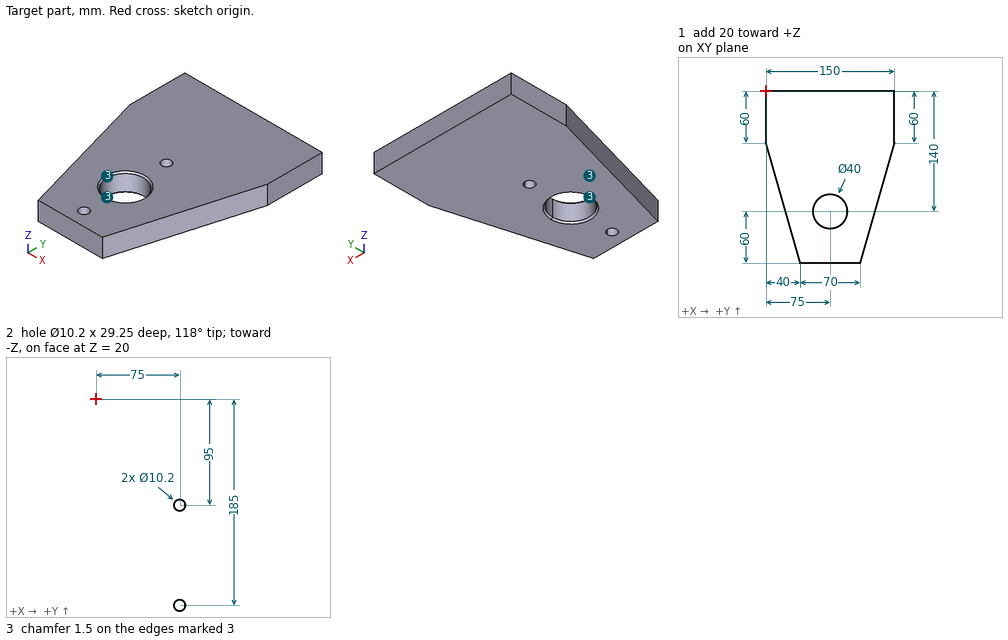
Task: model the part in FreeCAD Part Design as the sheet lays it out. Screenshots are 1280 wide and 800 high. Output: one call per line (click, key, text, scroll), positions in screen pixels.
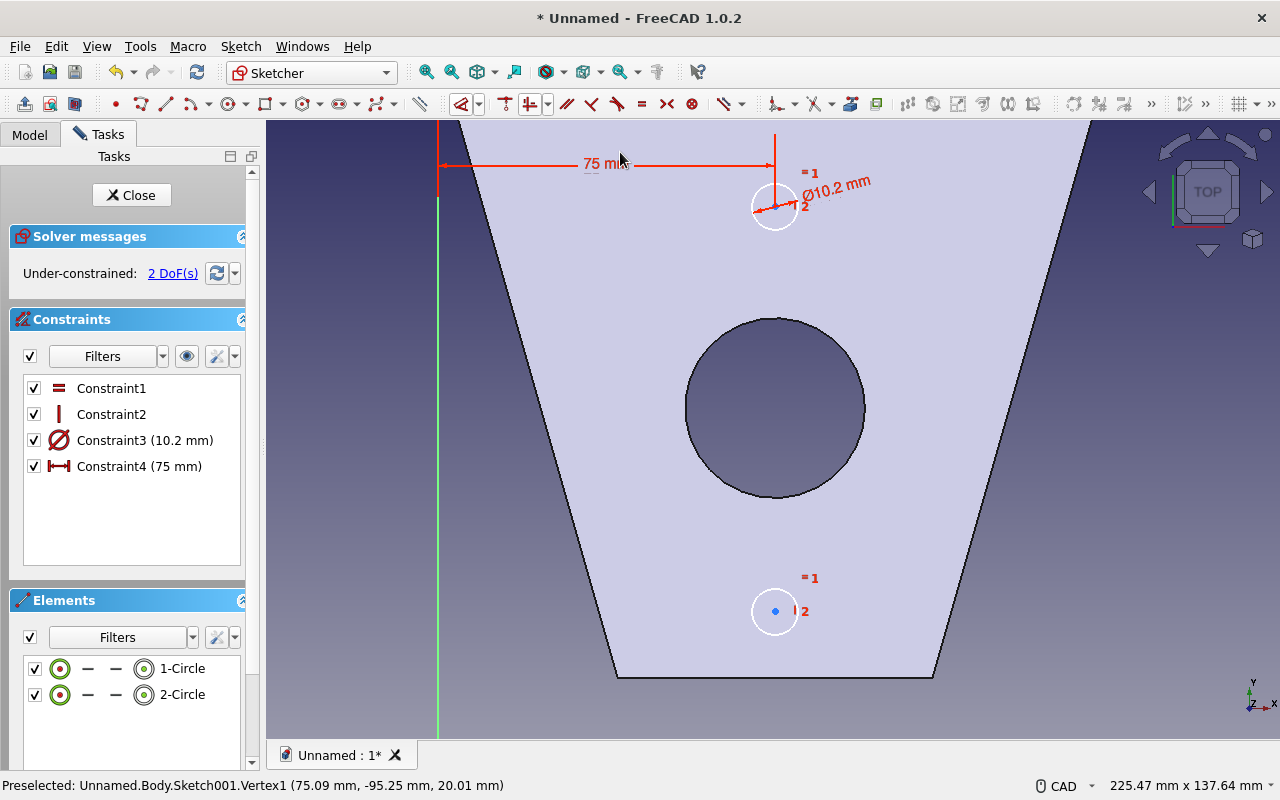
click(775, 207)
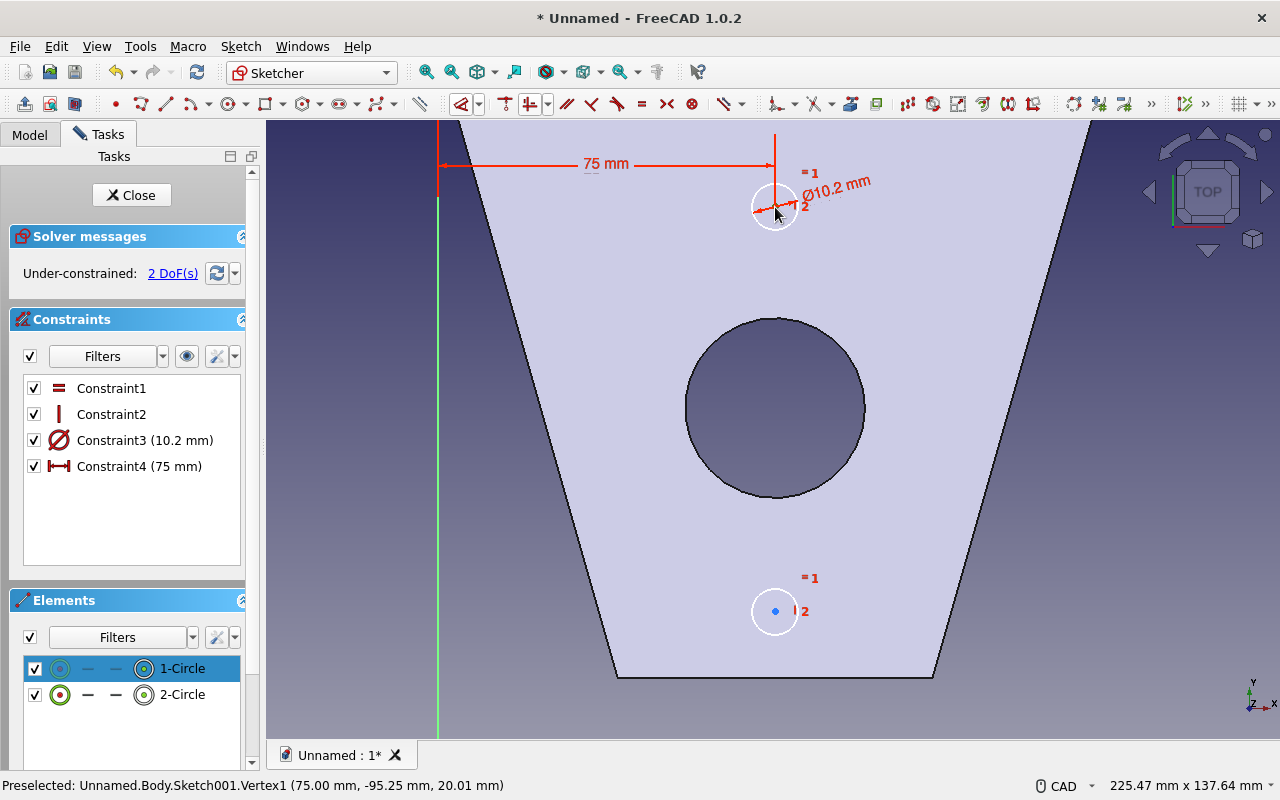
click(478, 104)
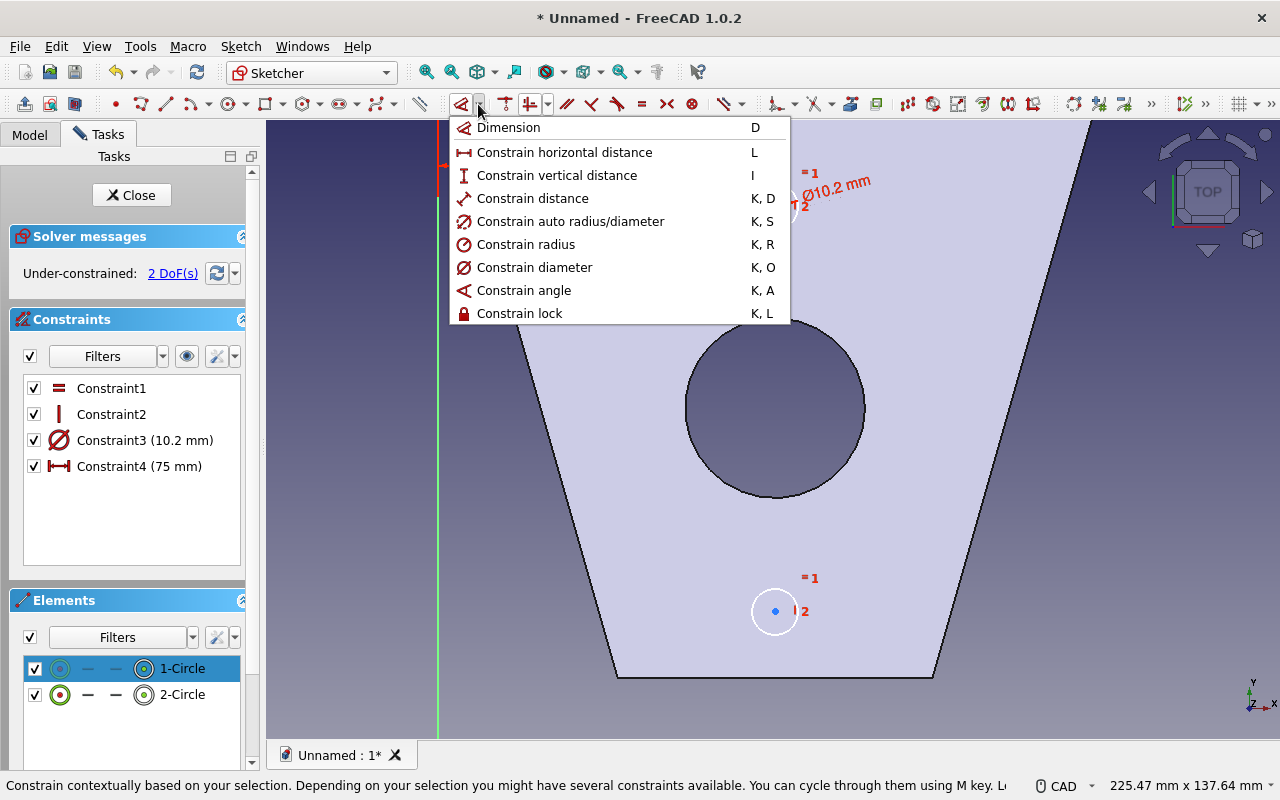
click(620, 176)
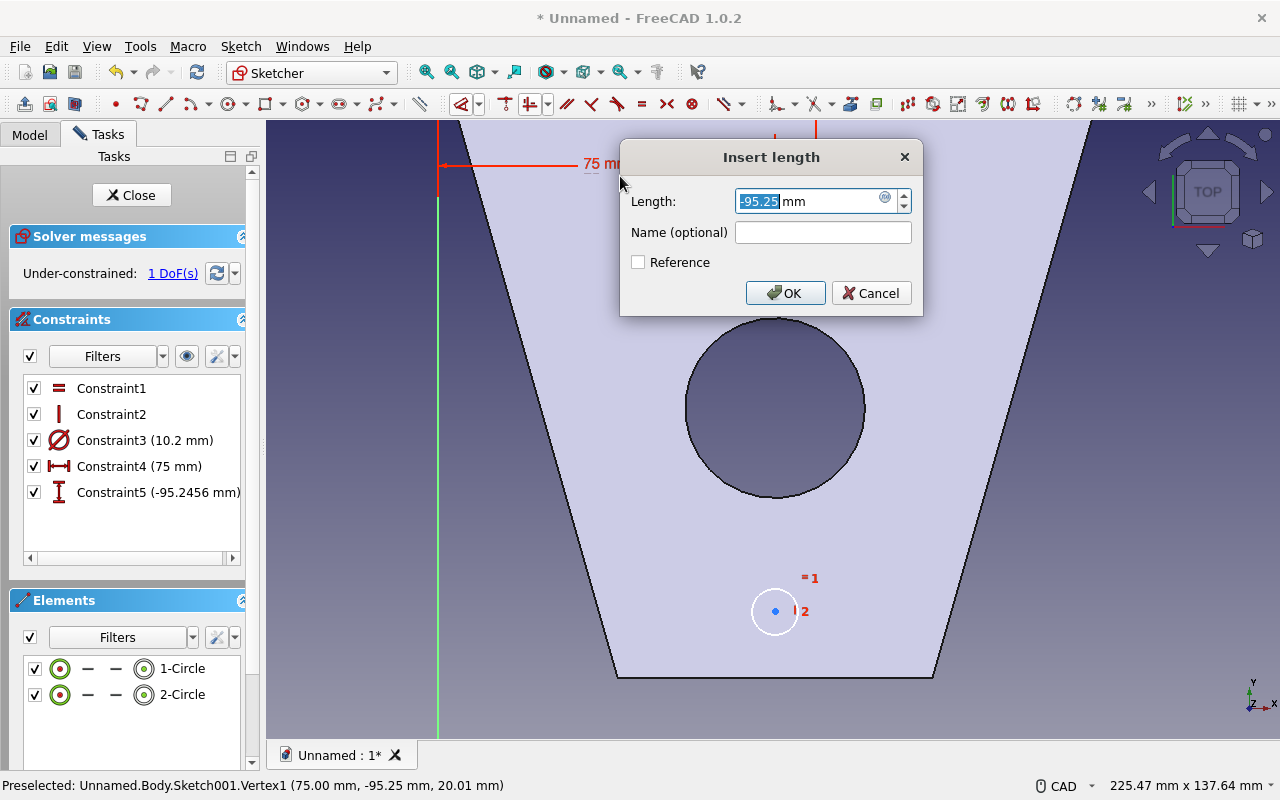
text(-95)
key(Return)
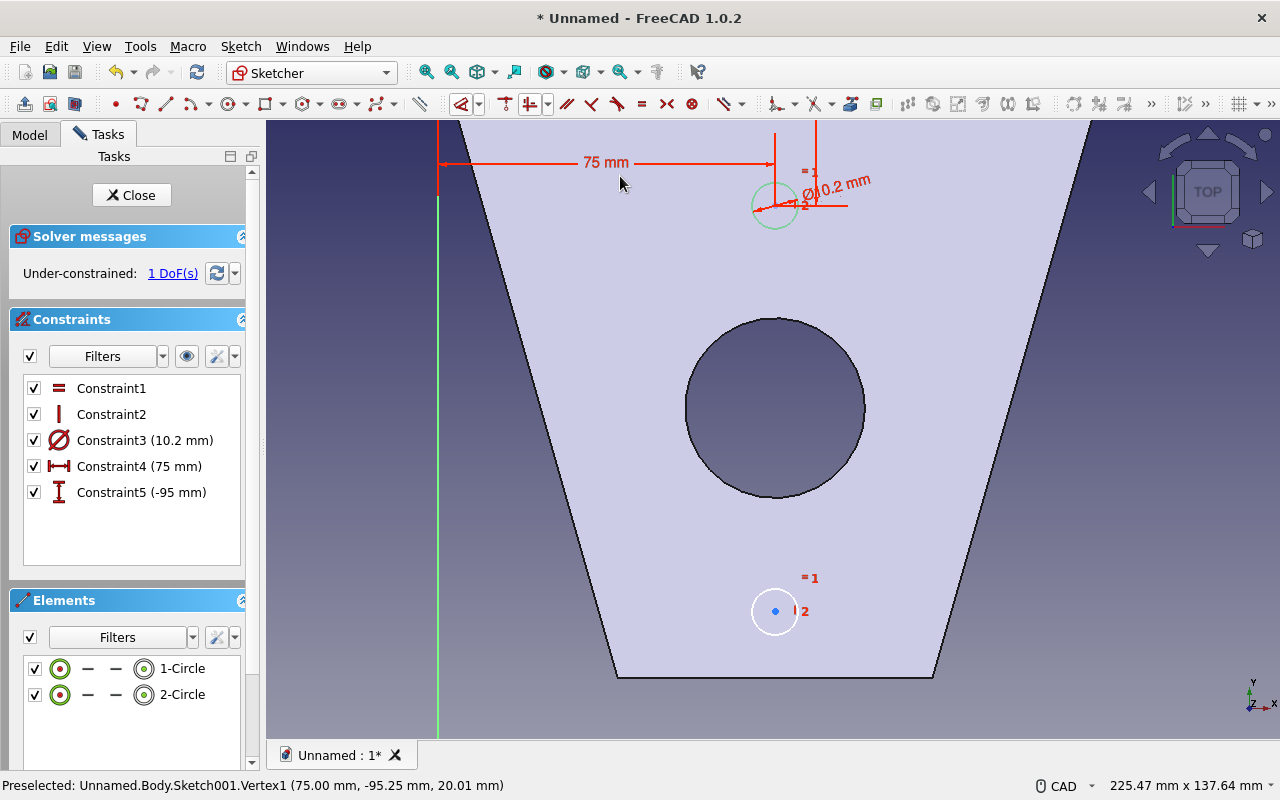
click(775, 612)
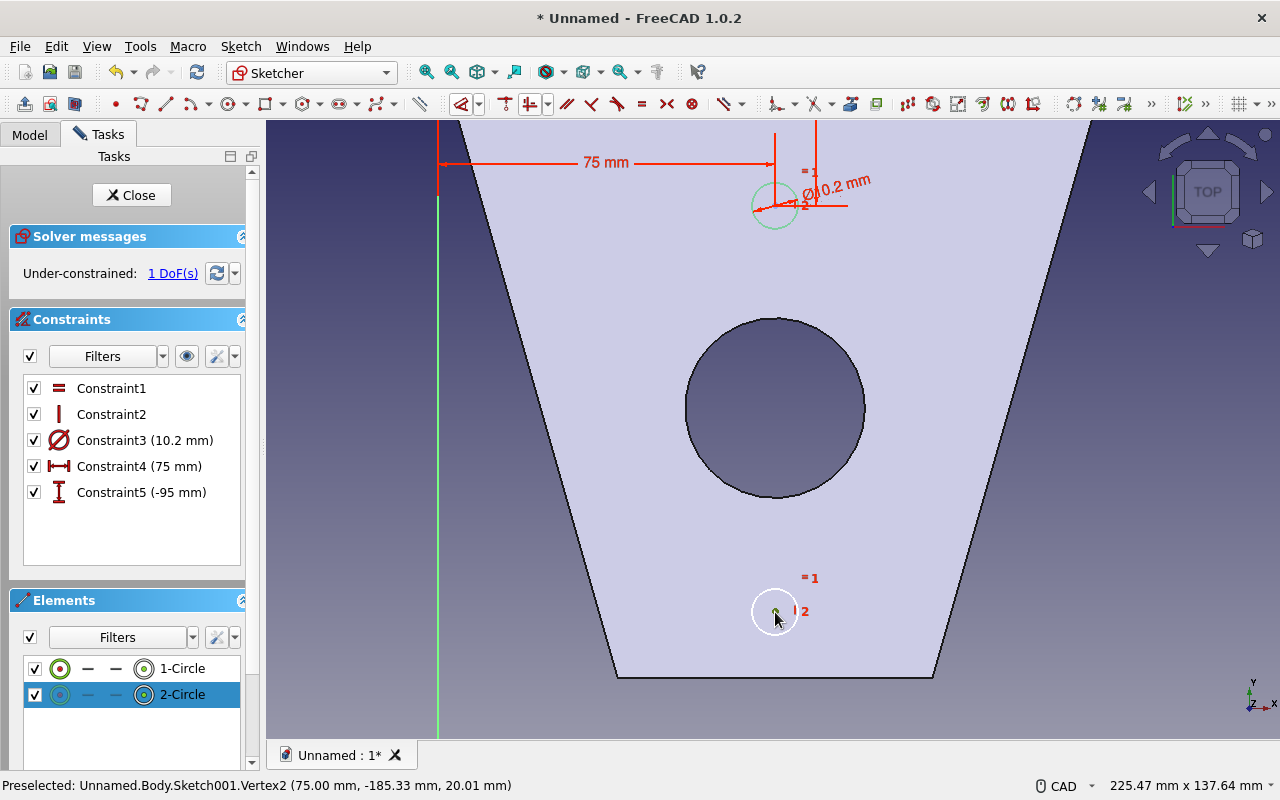
key(i)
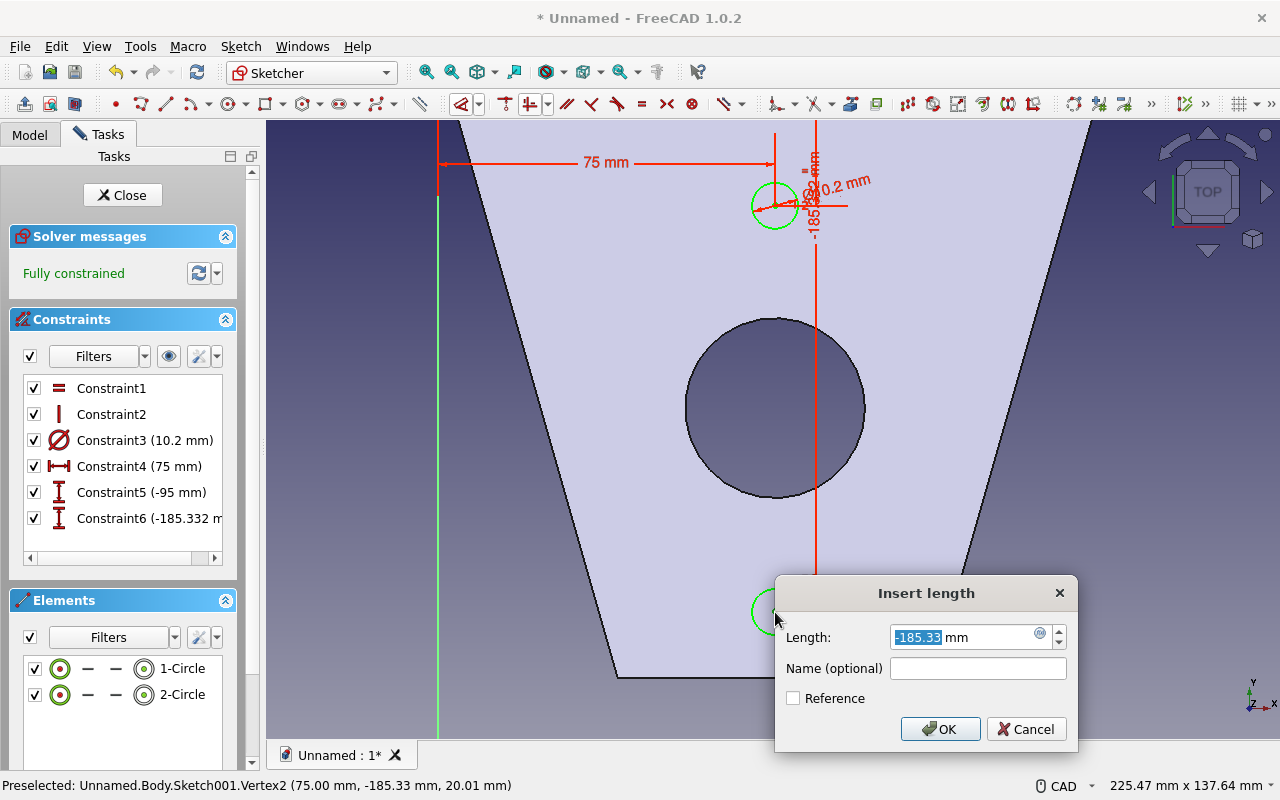
text(-185)
key(Return)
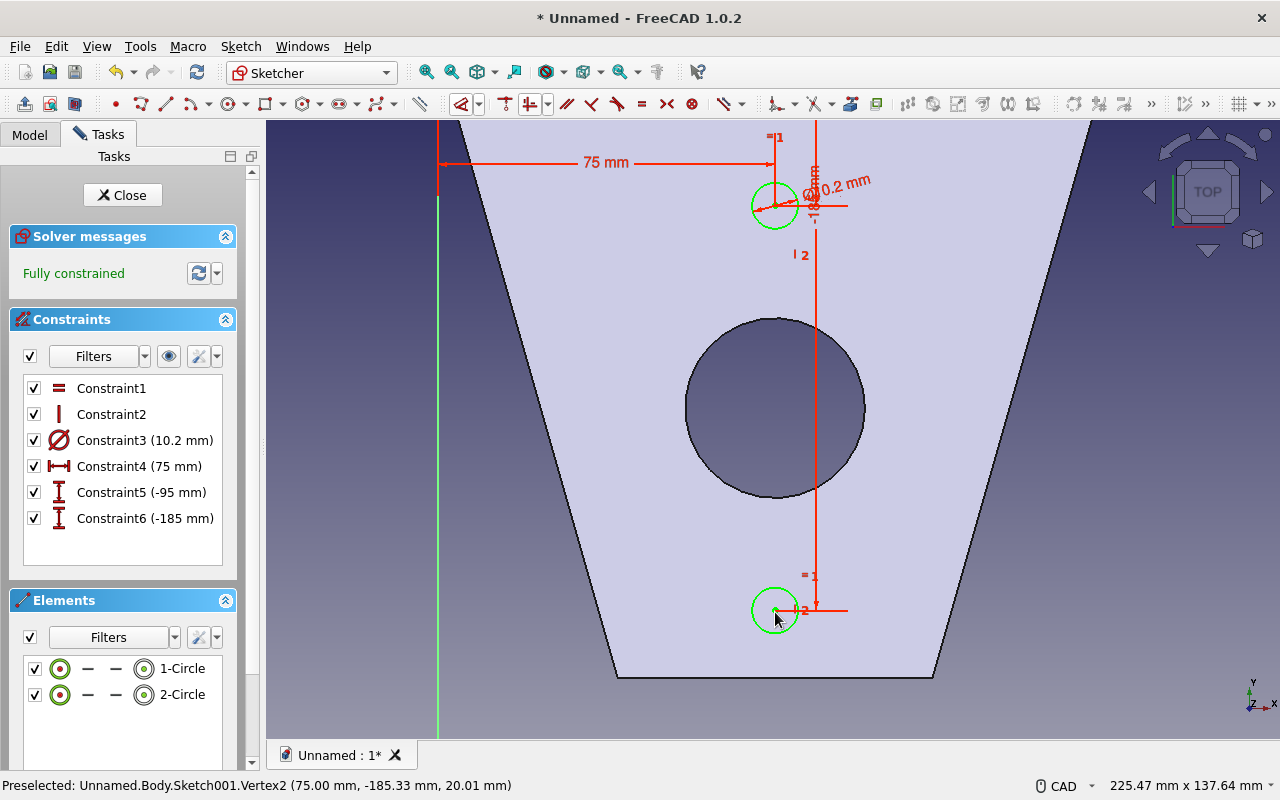
click(123, 195)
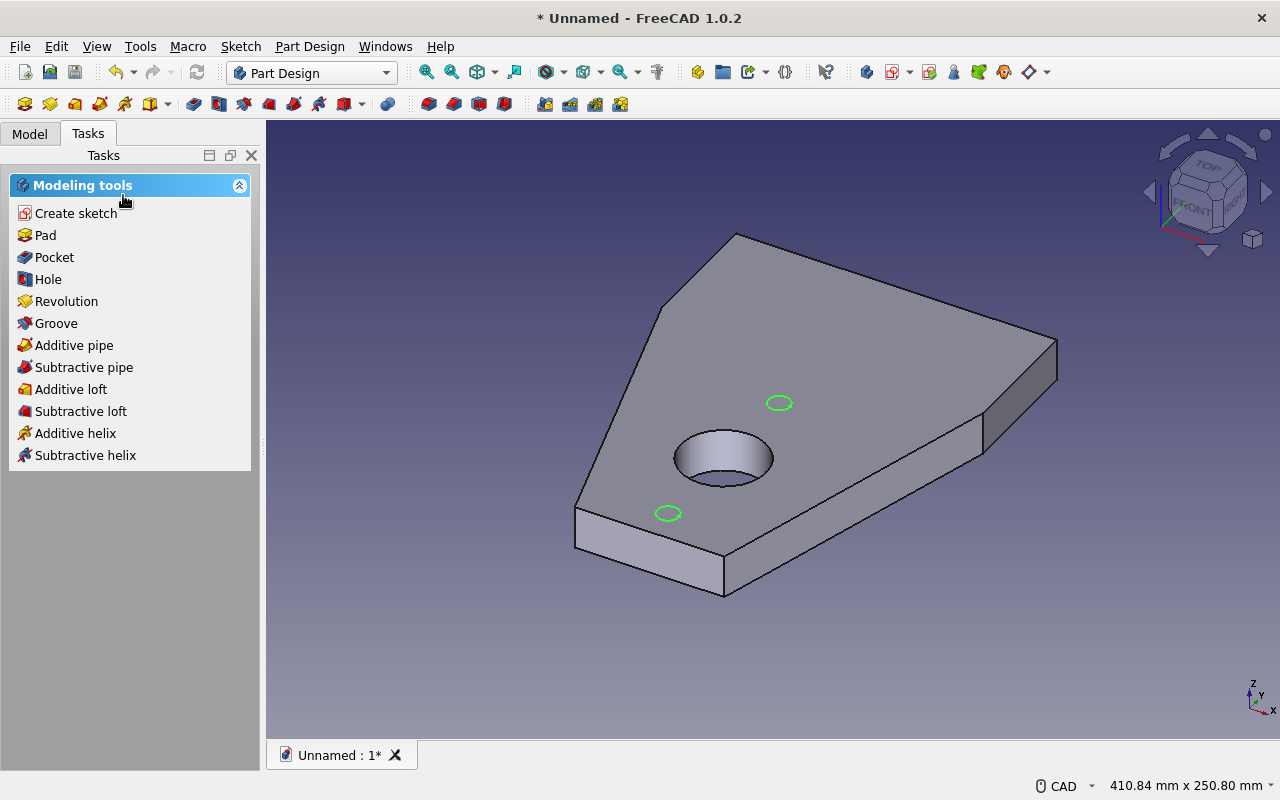
click(219, 104)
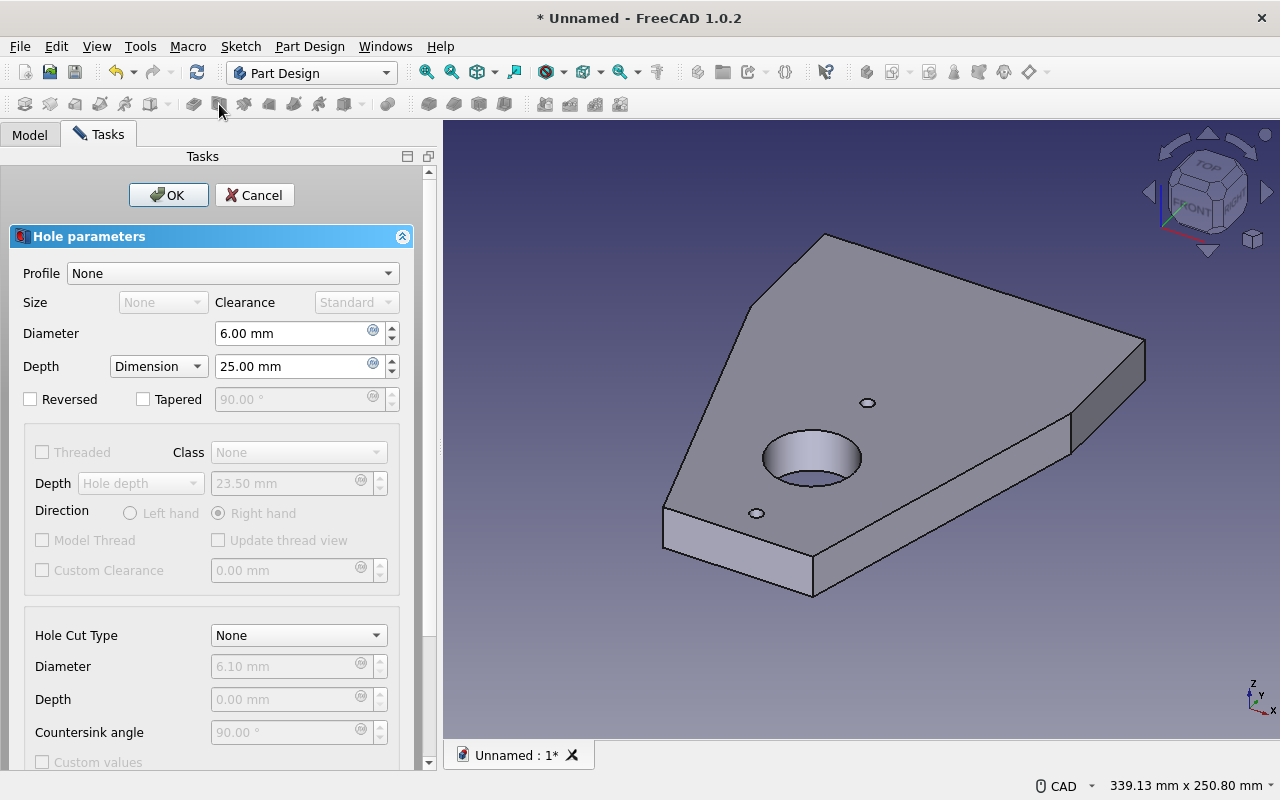
triple_click(300, 334)